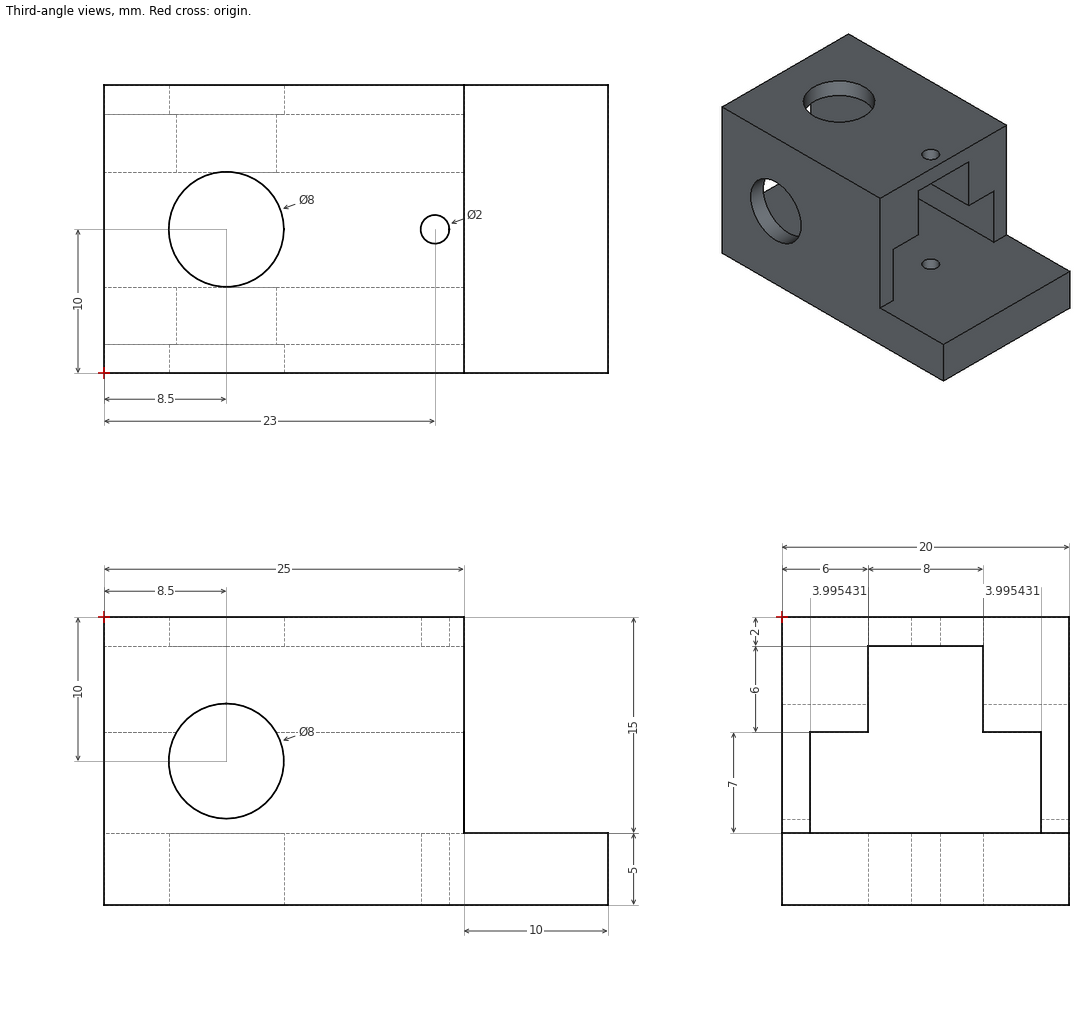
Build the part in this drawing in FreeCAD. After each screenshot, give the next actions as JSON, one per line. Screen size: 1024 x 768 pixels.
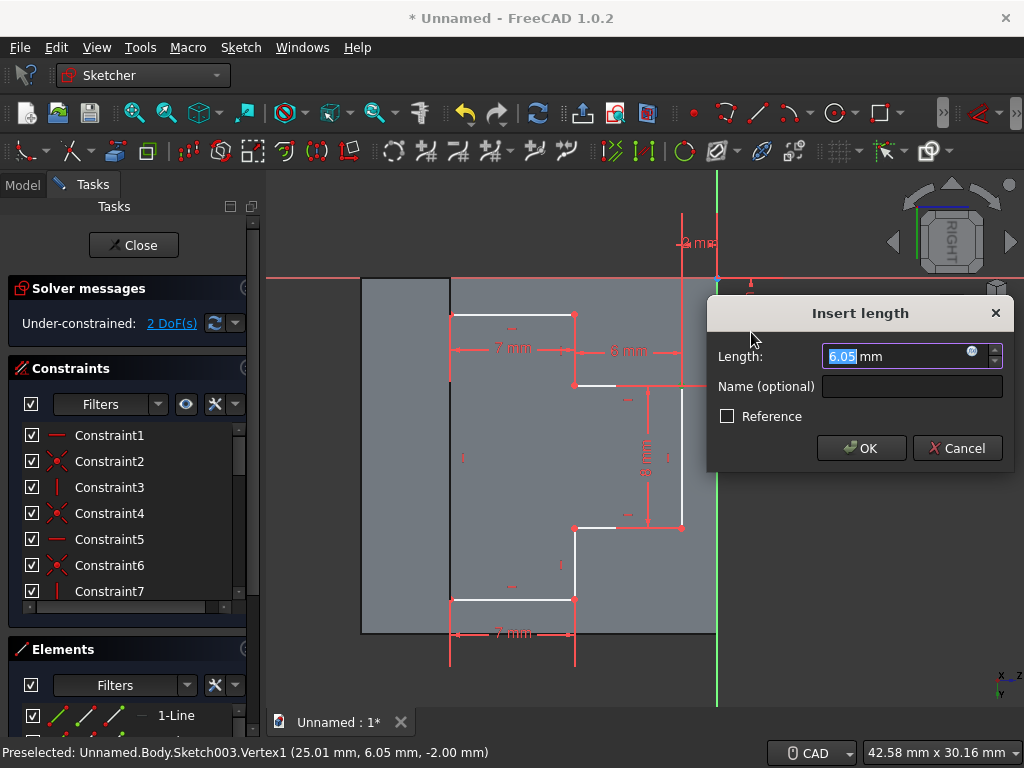
{"action": "type", "text": "6"}
{"action": "key", "text": "Return"}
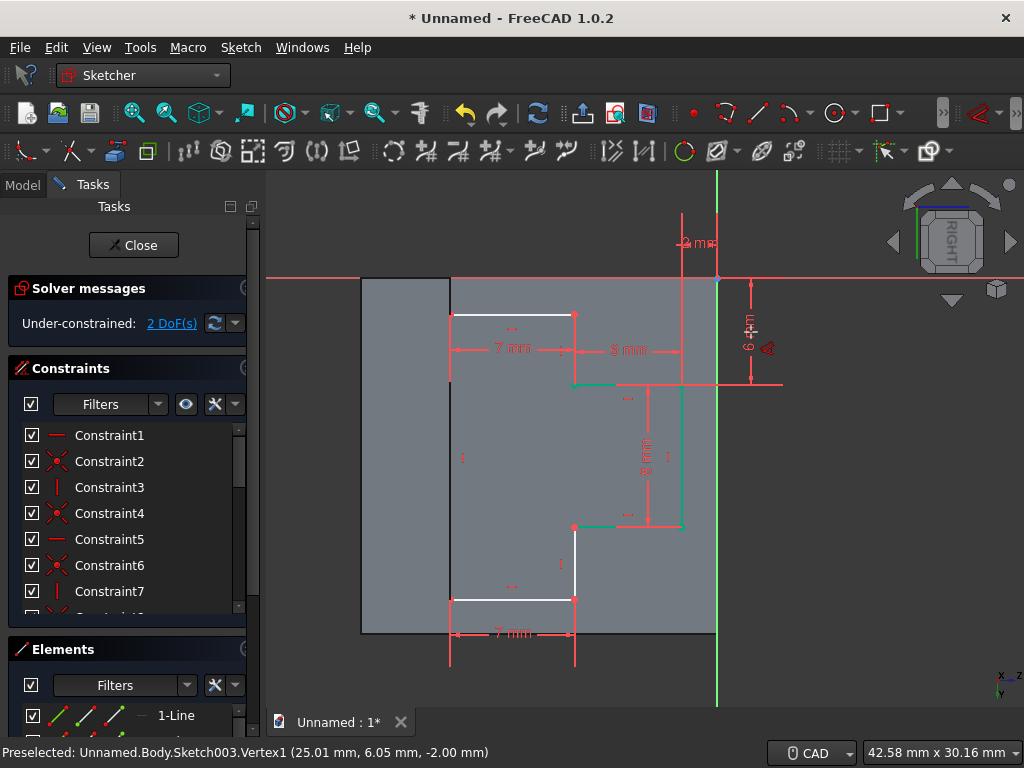
{"action": "left_click", "coordinate": [575, 364]}
{"action": "left_click", "coordinate": [541, 375]}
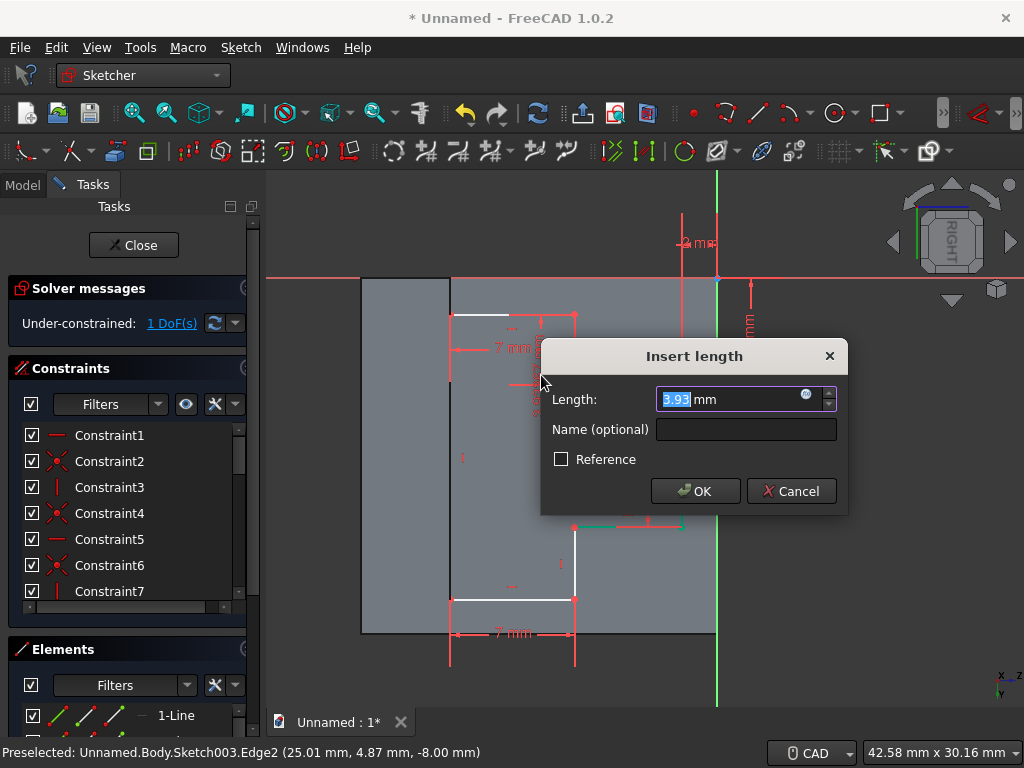
{"action": "type", "text": "3.995431"}
{"action": "key", "text": "Return"}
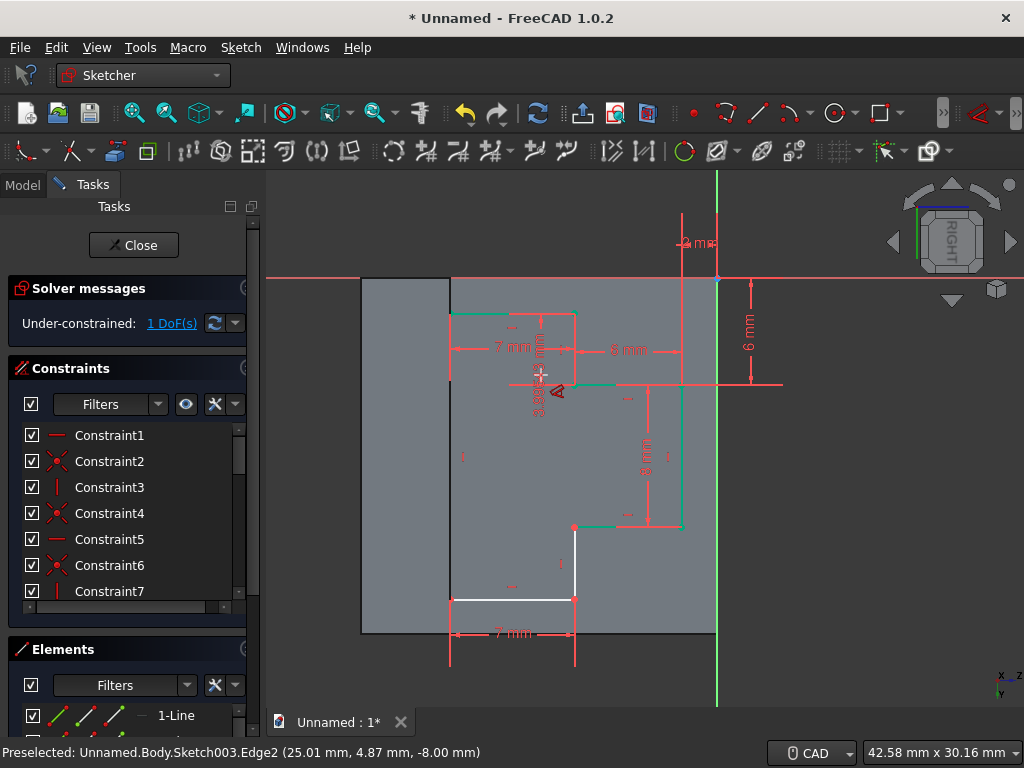
{"action": "left_click", "coordinate": [575, 578]}
{"action": "left_click", "coordinate": [541, 564]}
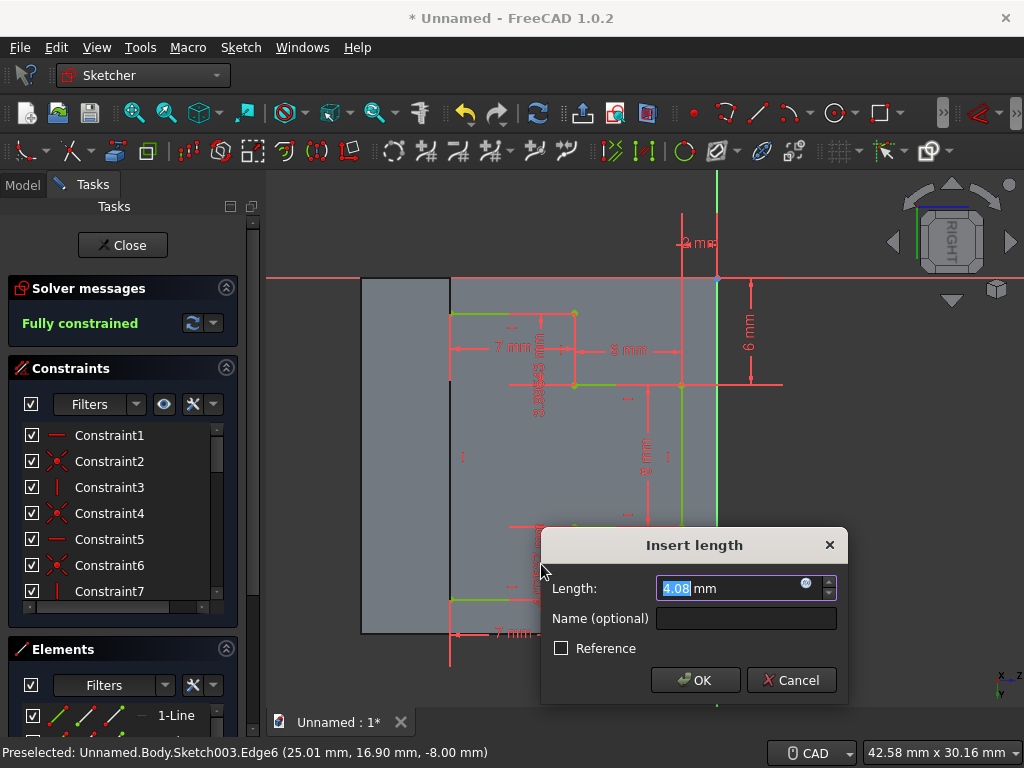
{"action": "type", "text": "3.995431"}
{"action": "key", "text": "Return"}
{"action": "key", "text": "Escape"}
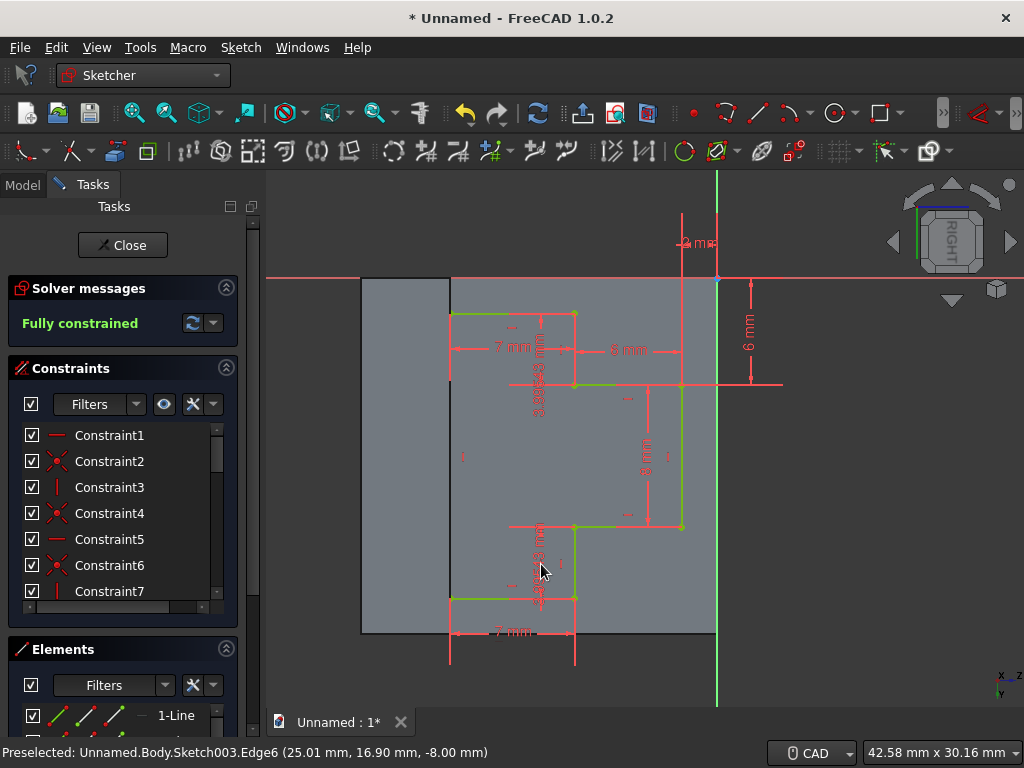
{"action": "left_click", "coordinate": [123, 245]}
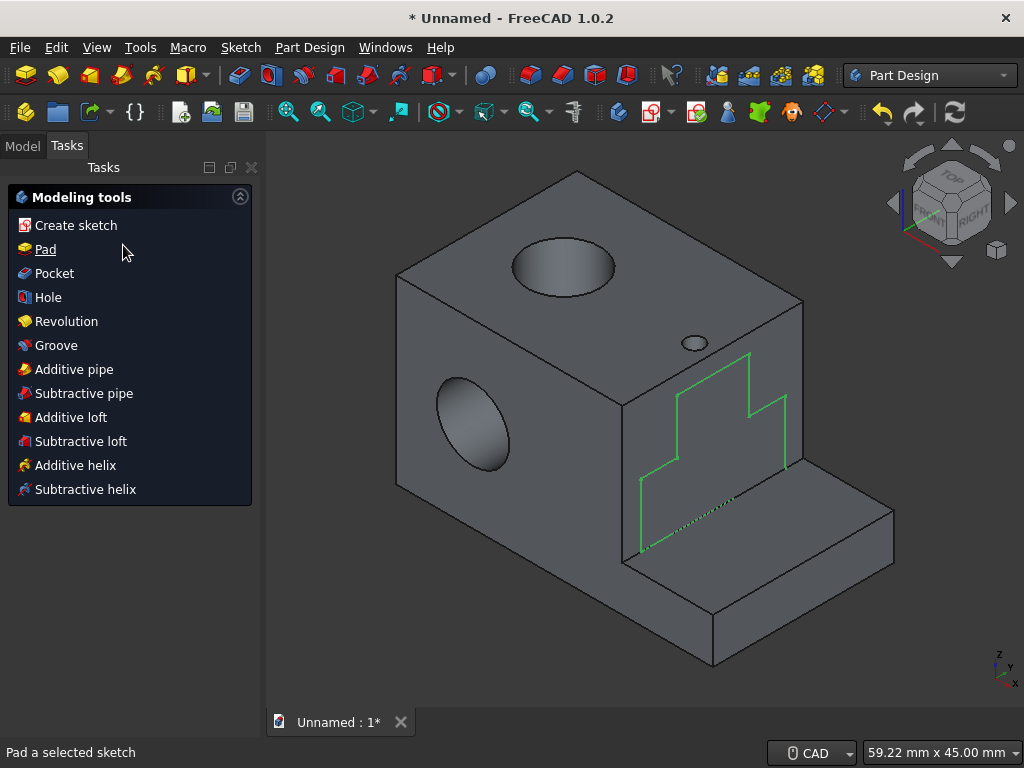
{"action": "left_click", "coordinate": [240, 76]}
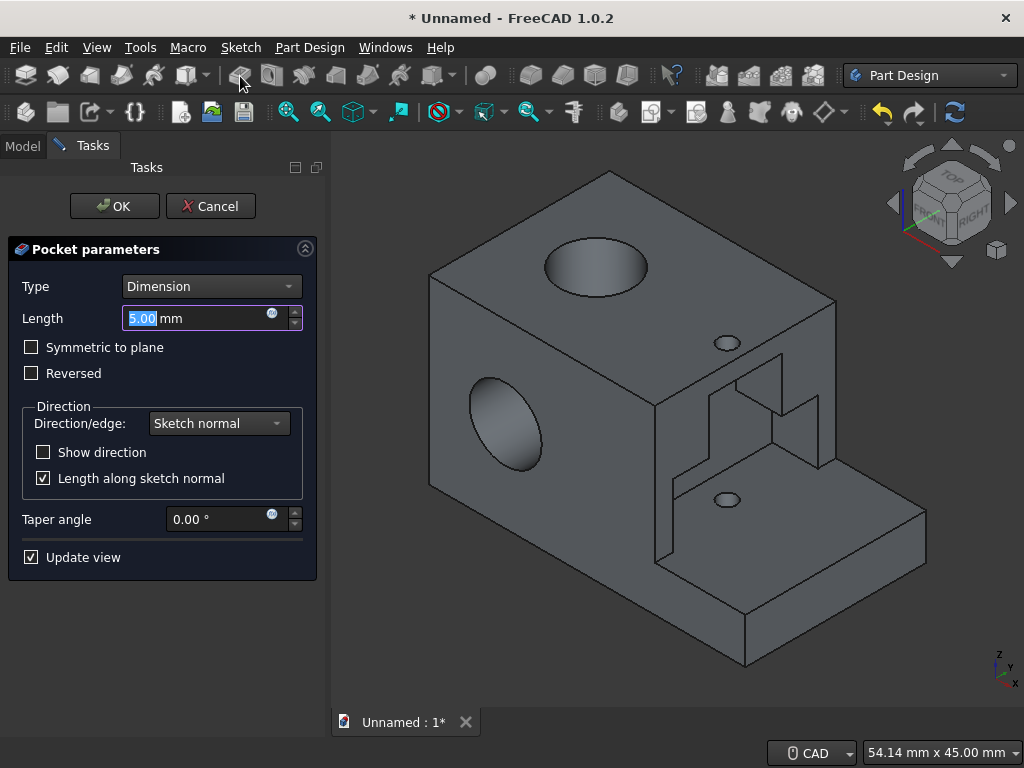
{"action": "left_click", "coordinate": [212, 286]}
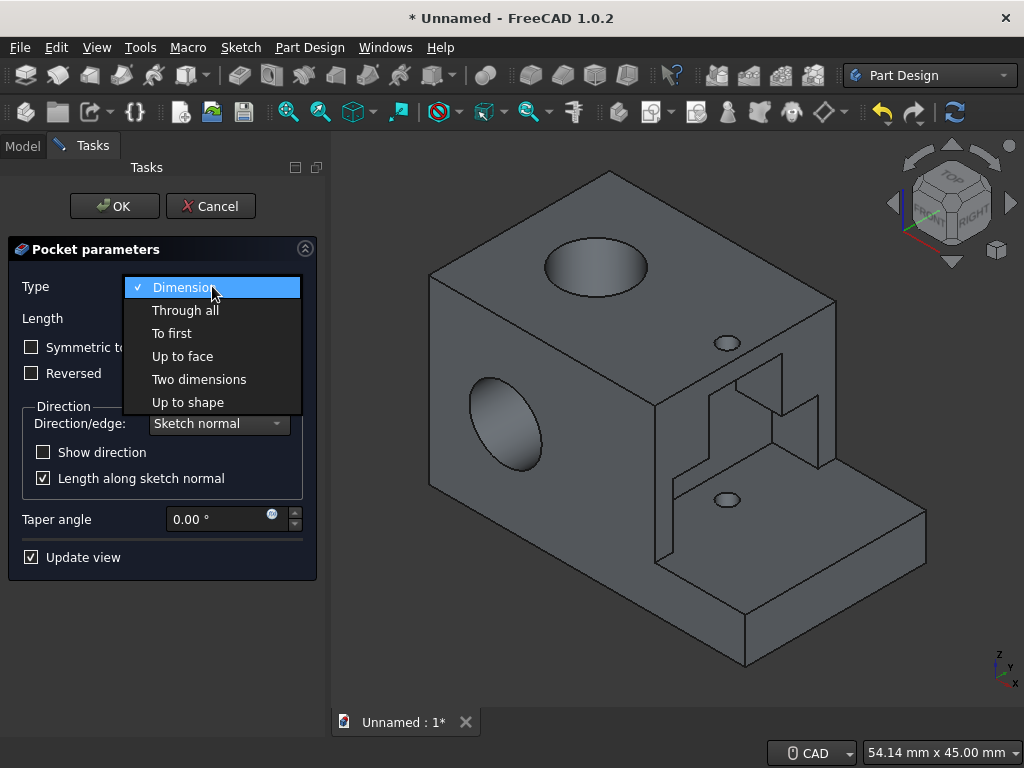
{"action": "left_click", "coordinate": [212, 310]}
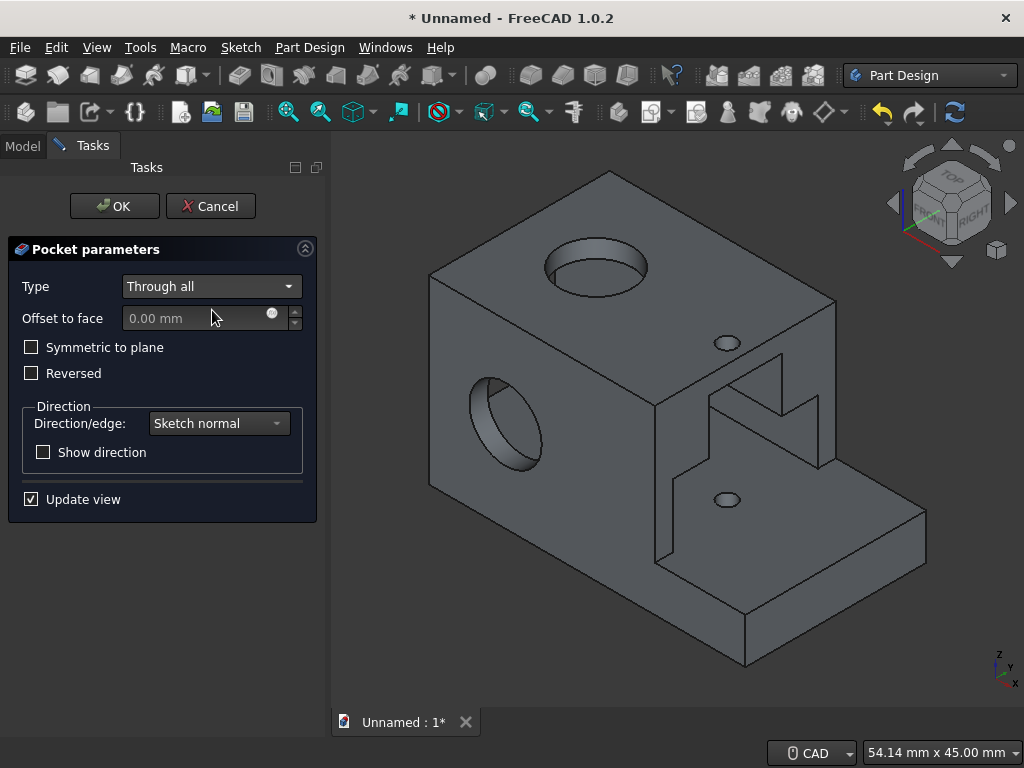
{"action": "left_click", "coordinate": [115, 206]}